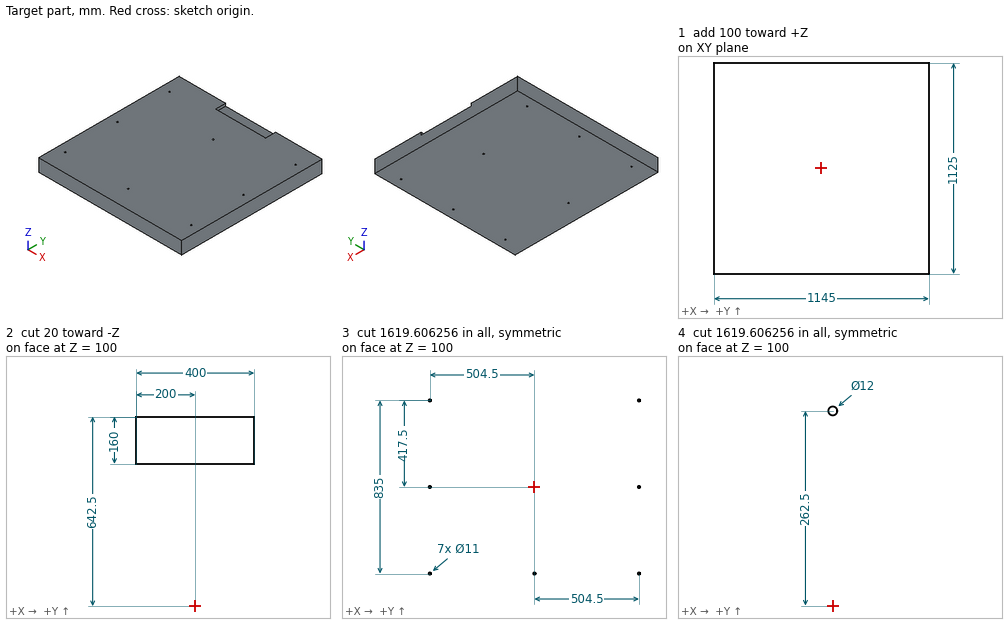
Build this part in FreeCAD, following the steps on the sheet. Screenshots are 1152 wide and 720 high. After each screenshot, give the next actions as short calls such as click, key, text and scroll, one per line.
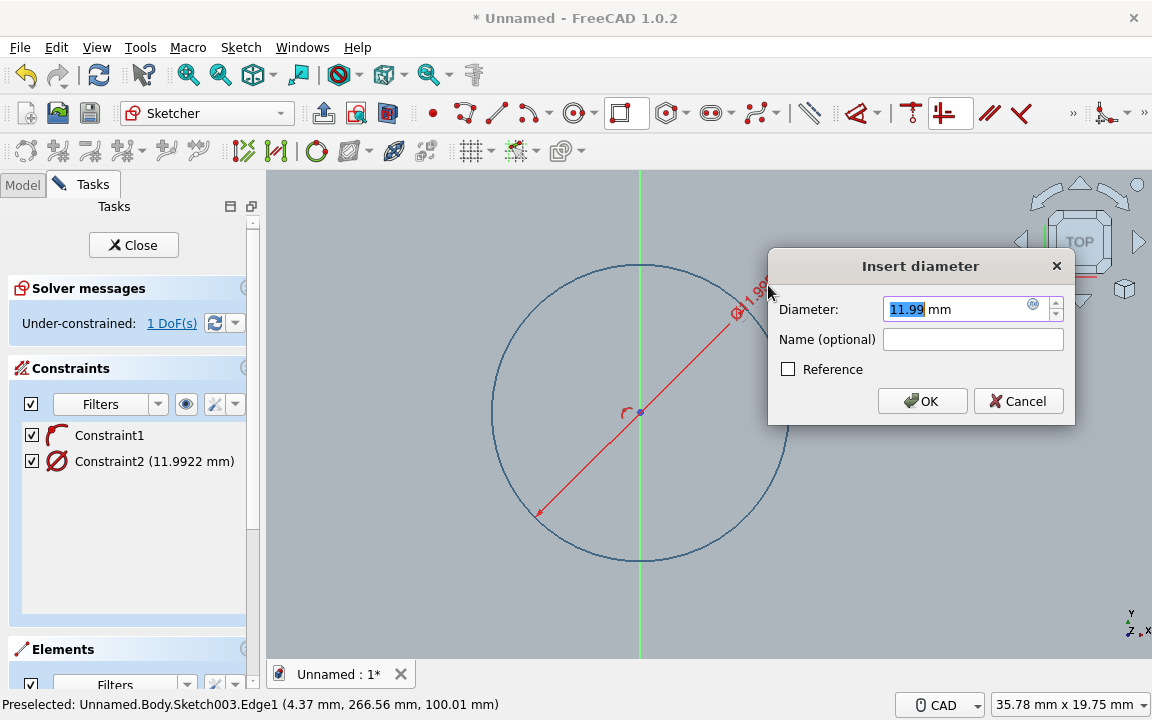
text(12)
key(Return)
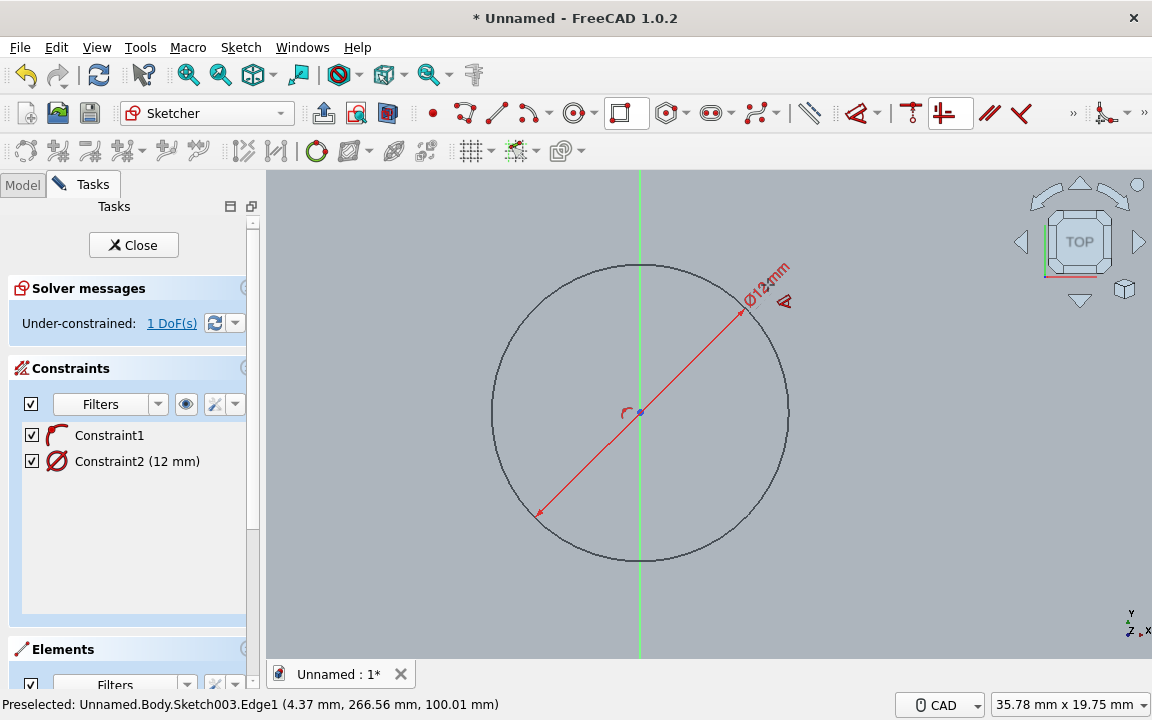
click(640, 413)
click(674, 522)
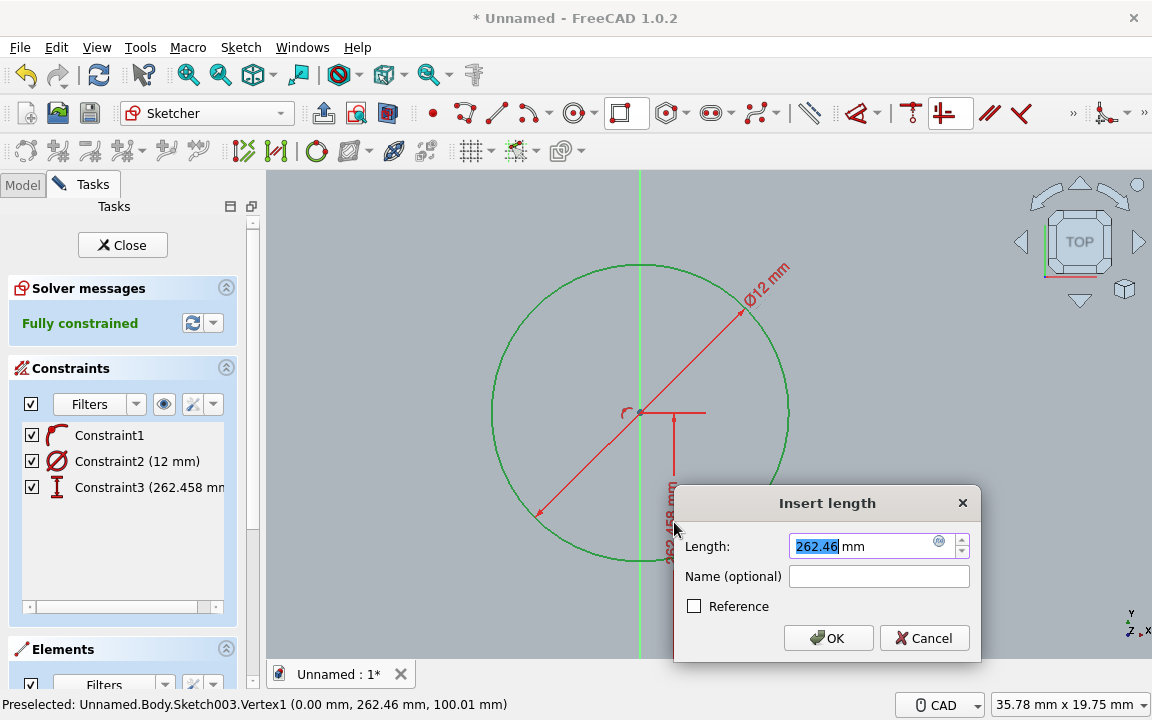
text(262.5)
key(Return)
key(Escape)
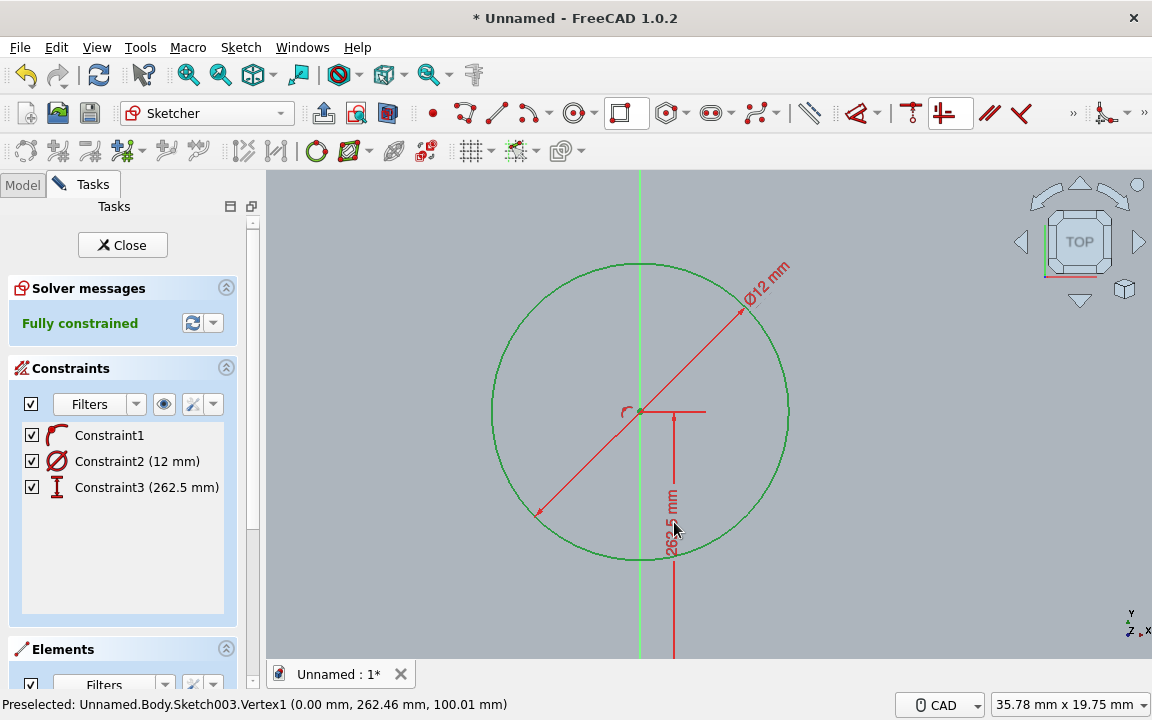
click(123, 245)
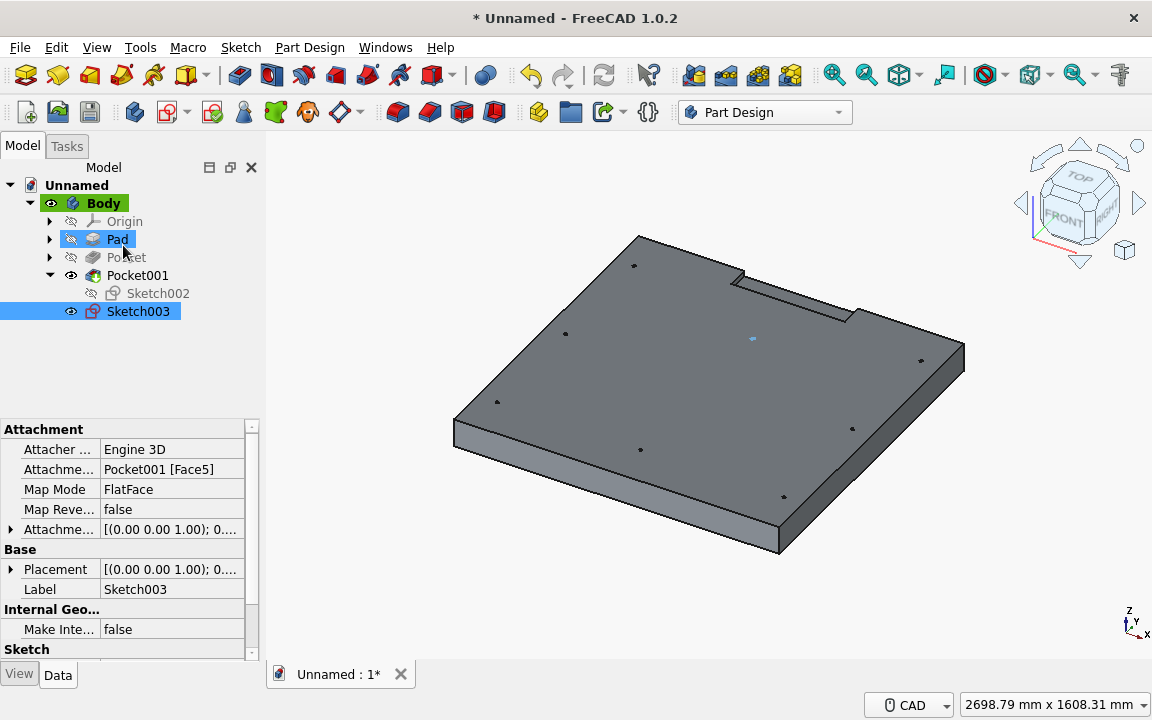
click(240, 76)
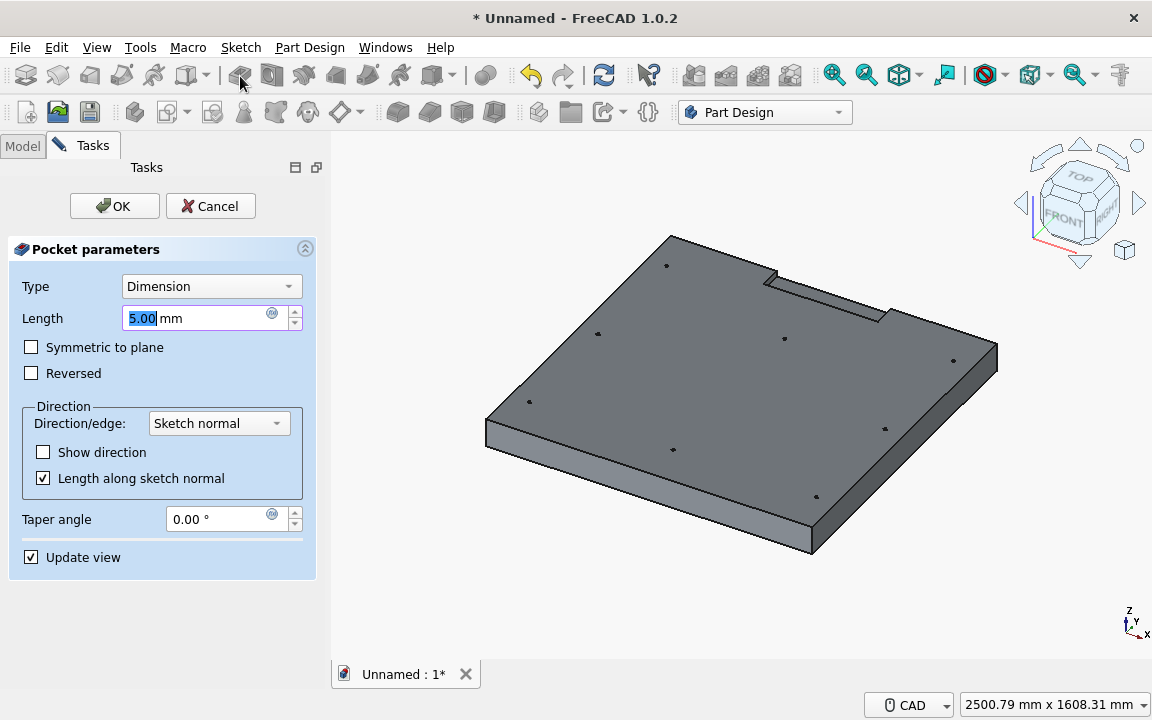
text(1619.606256)
key(Tab)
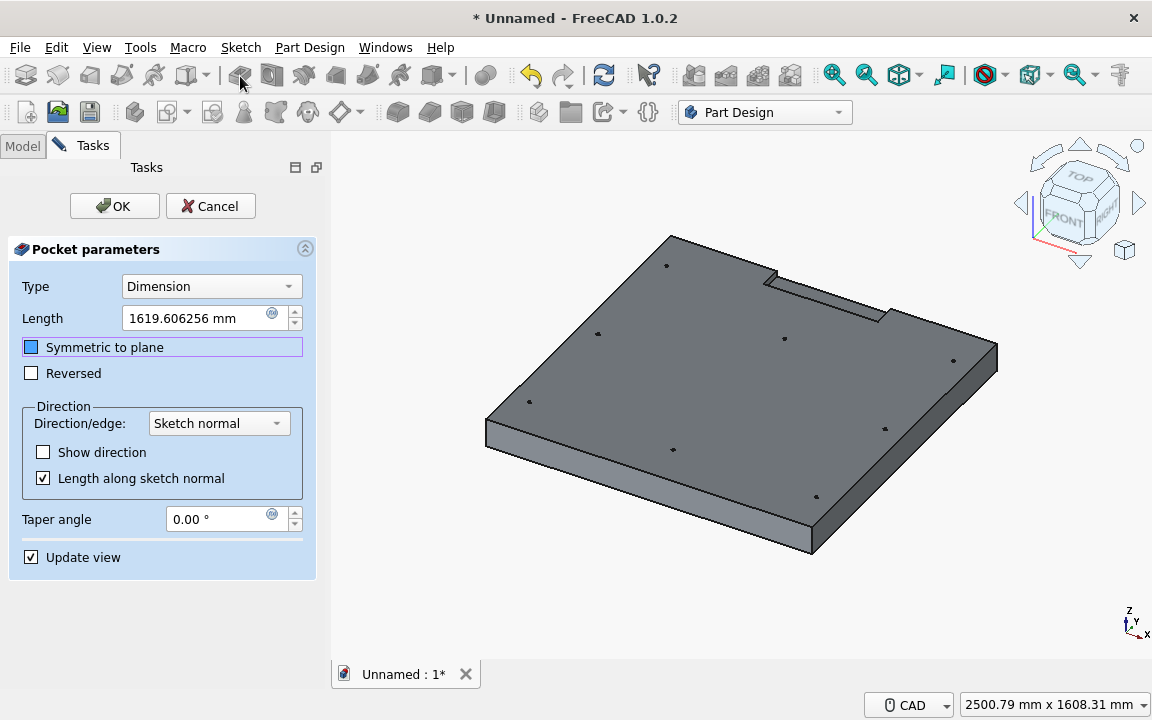
click(30, 347)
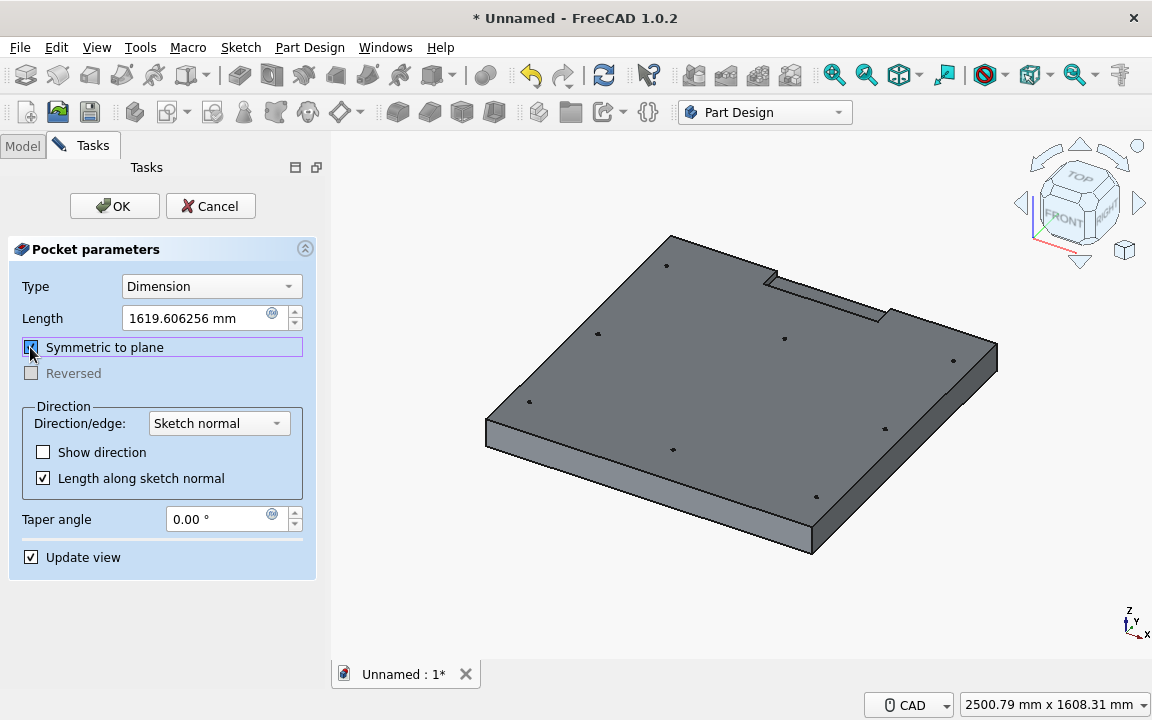
click(115, 206)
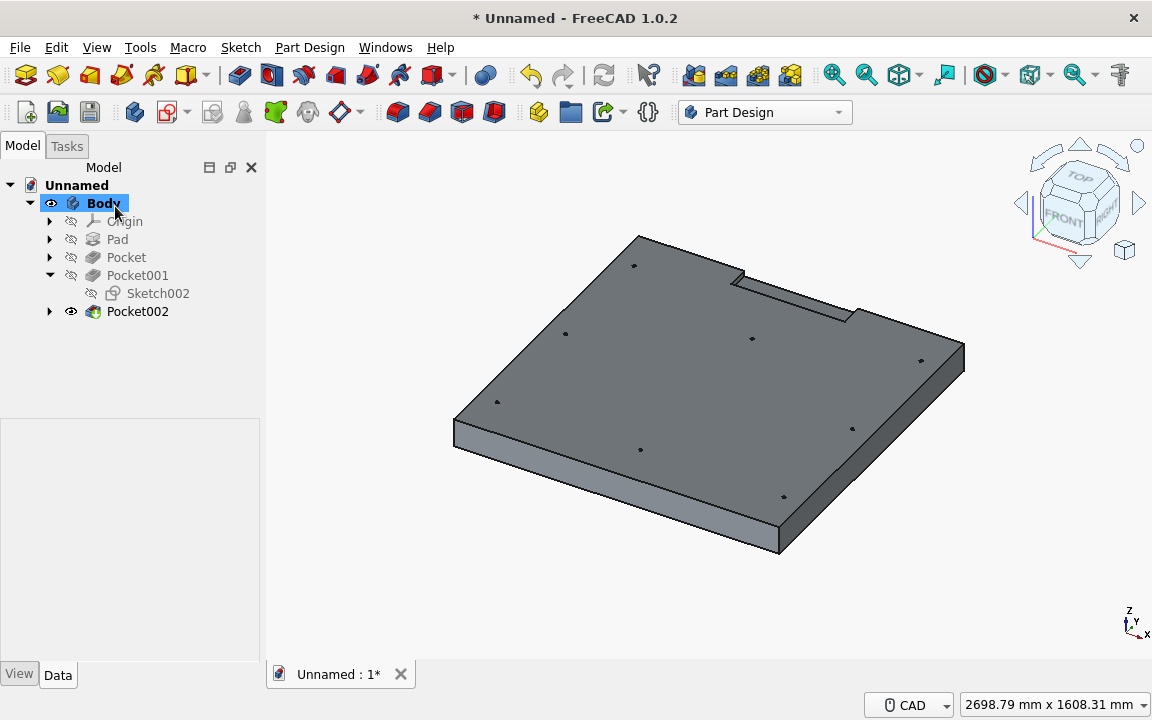
key(0)